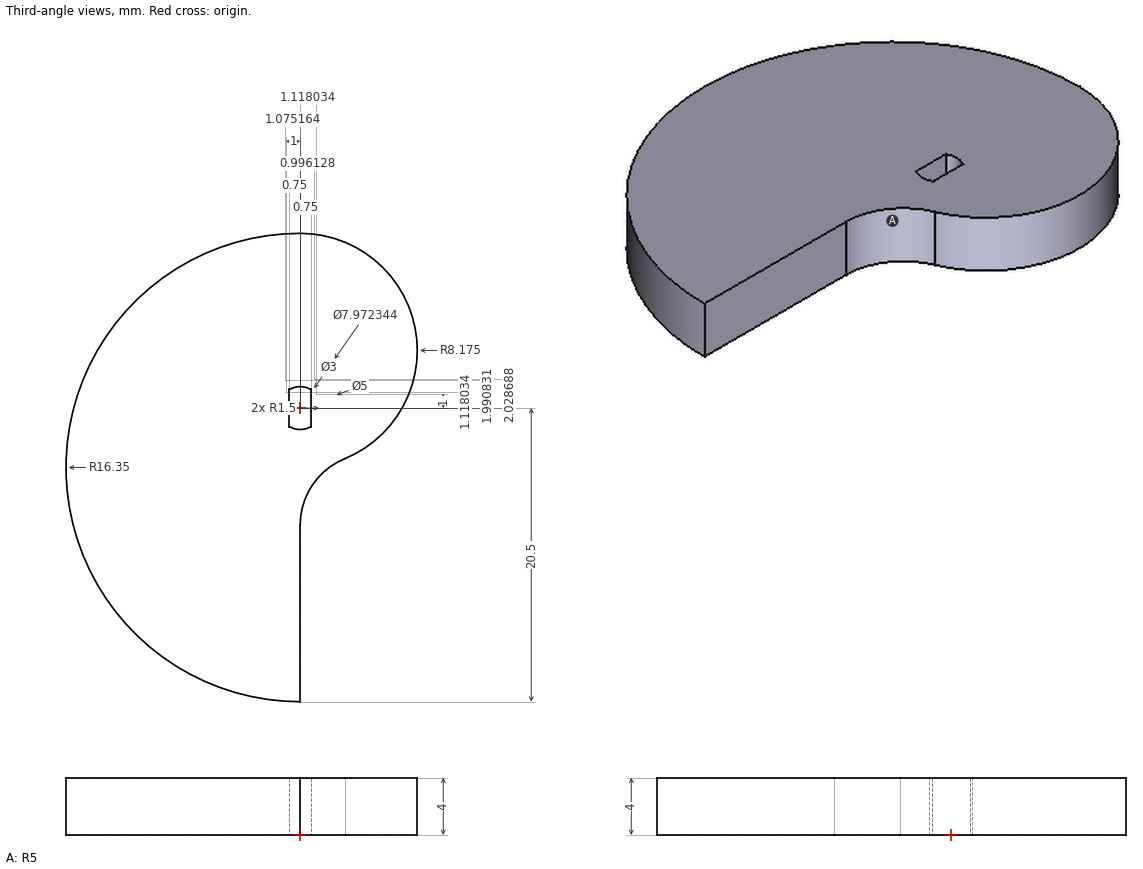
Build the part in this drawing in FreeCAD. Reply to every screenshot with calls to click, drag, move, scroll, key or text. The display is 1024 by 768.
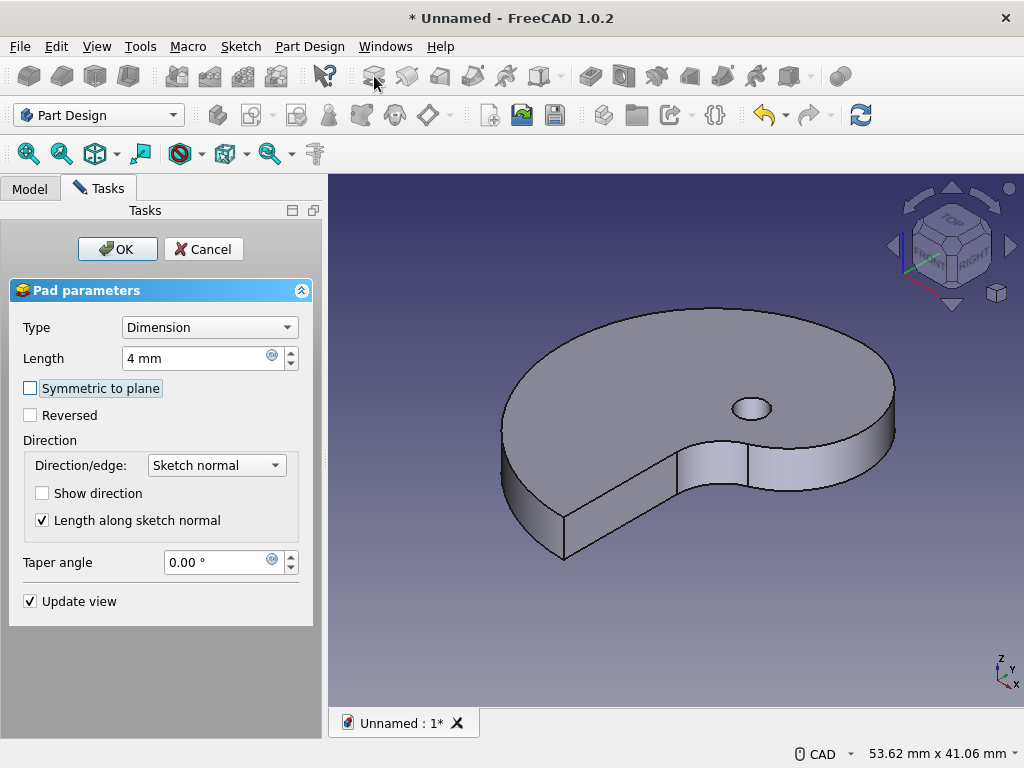
click(31, 415)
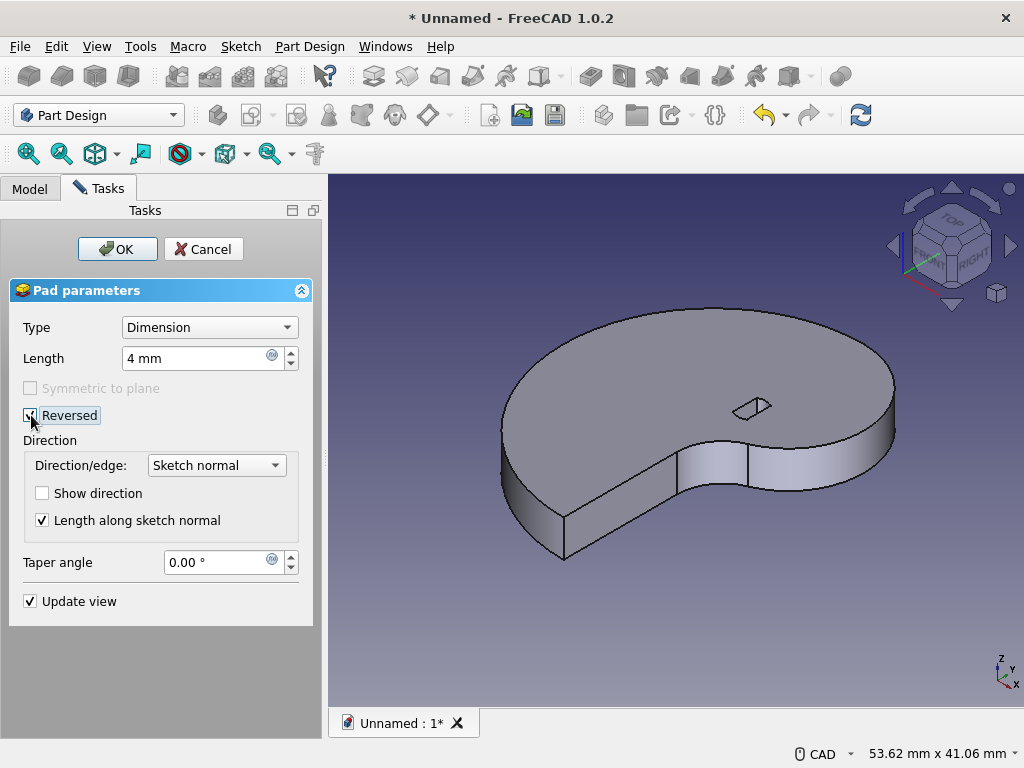
click(118, 249)